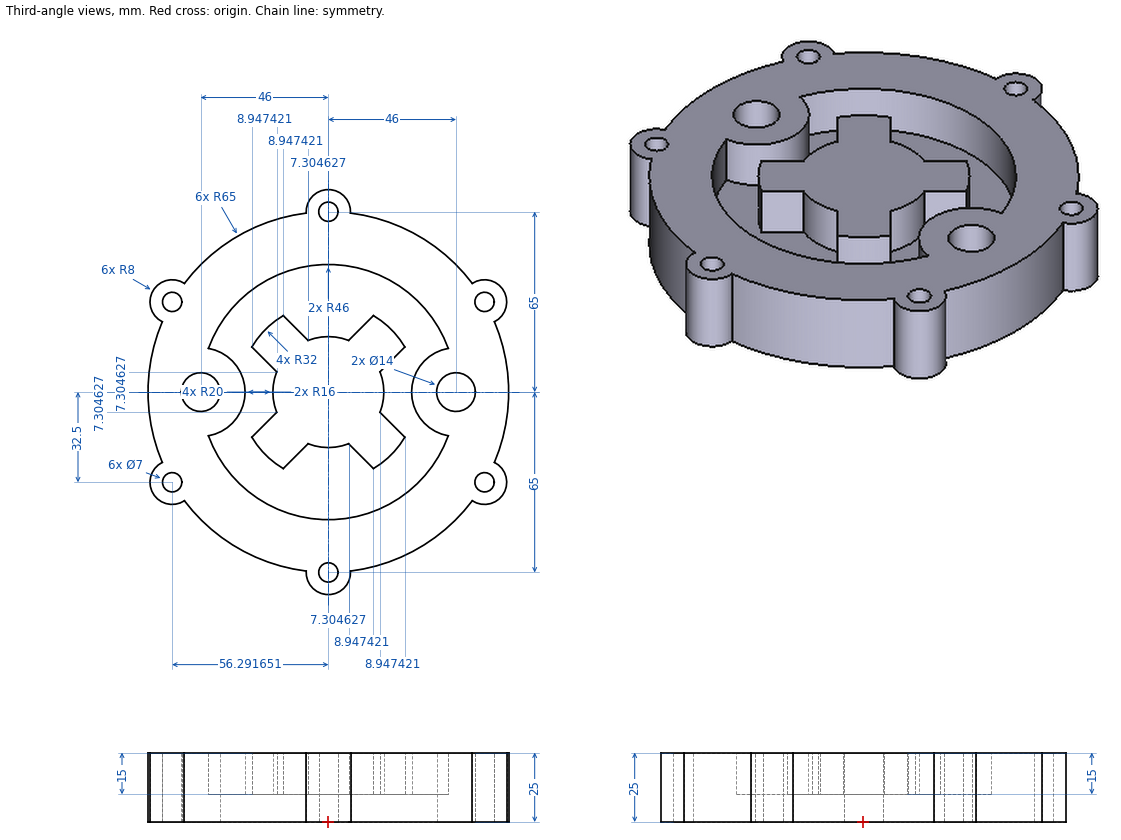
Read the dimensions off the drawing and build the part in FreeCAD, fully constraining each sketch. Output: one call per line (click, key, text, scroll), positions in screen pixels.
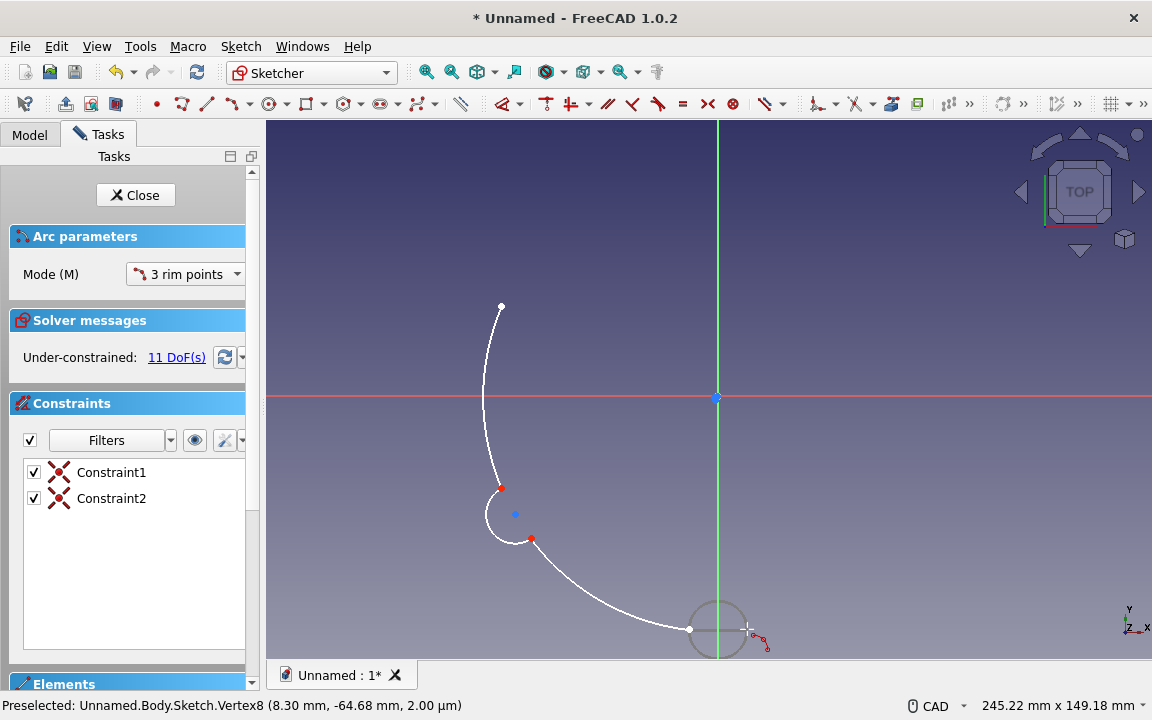
scroll(483, 376, down, 2)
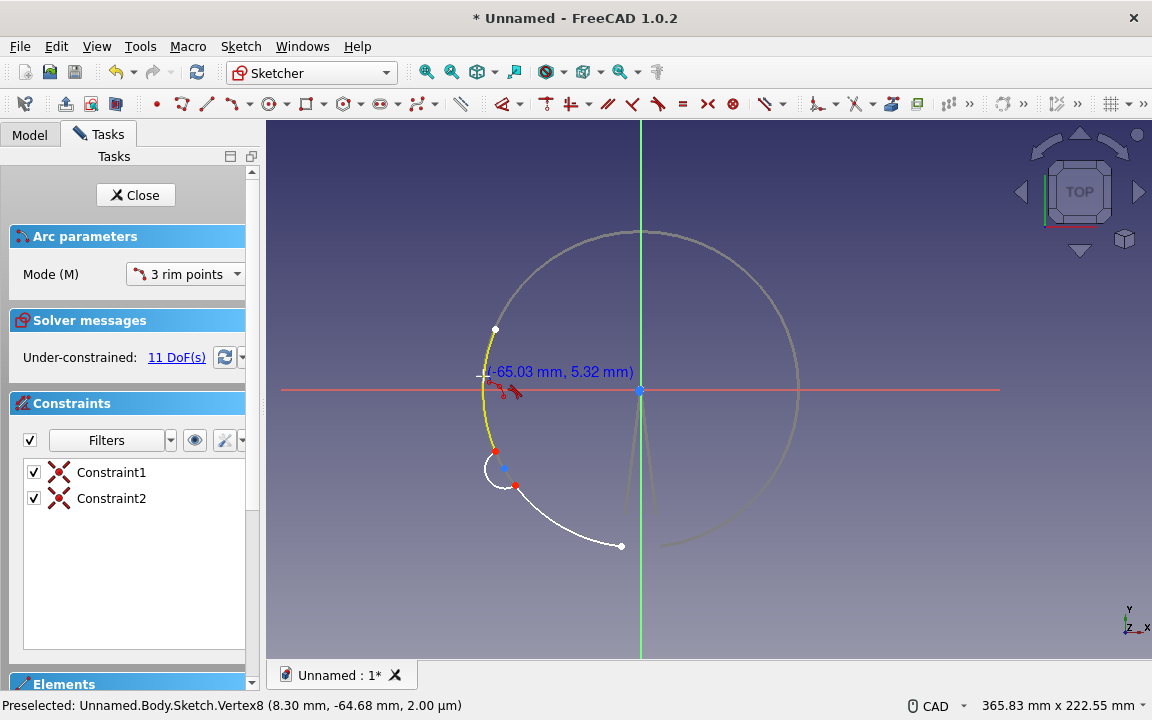
scroll(629, 563, up, 2)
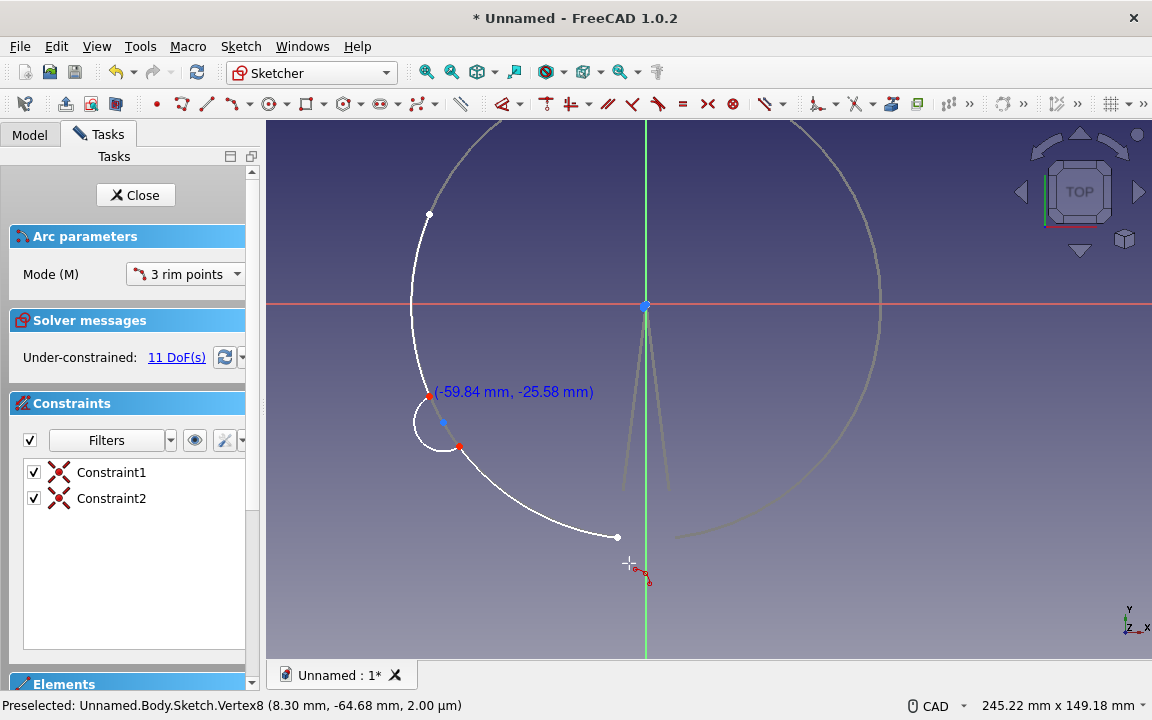
click(629, 562)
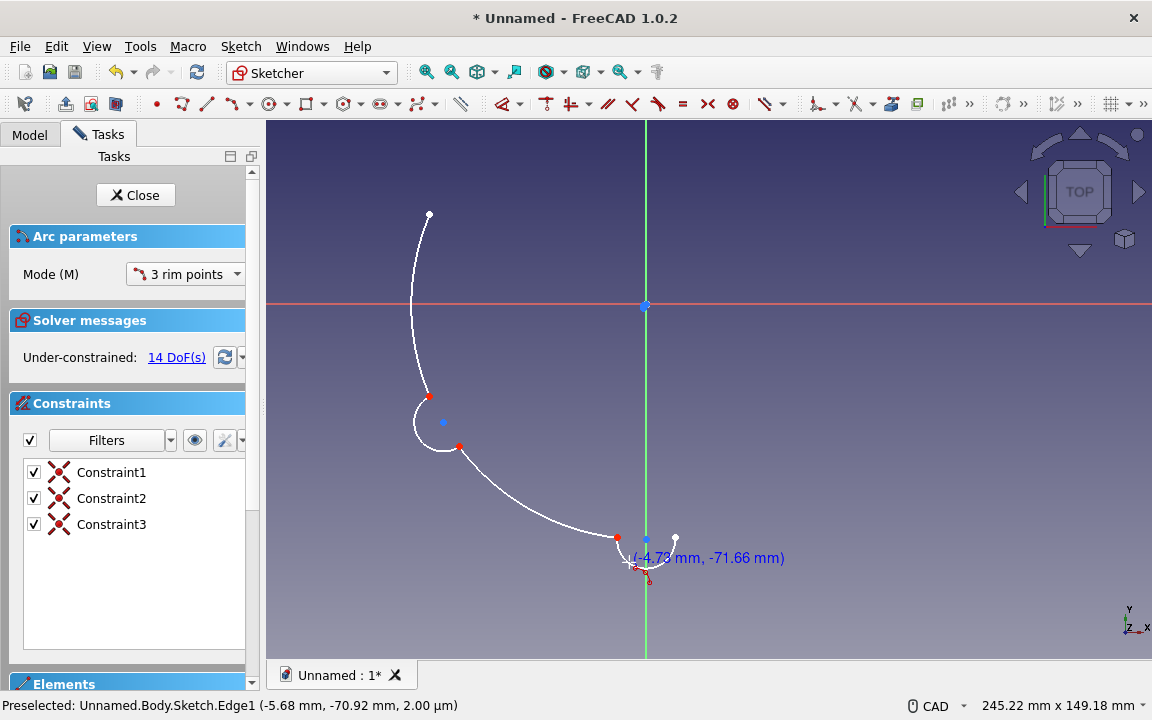
click(675, 538)
click(833, 446)
click(764, 507)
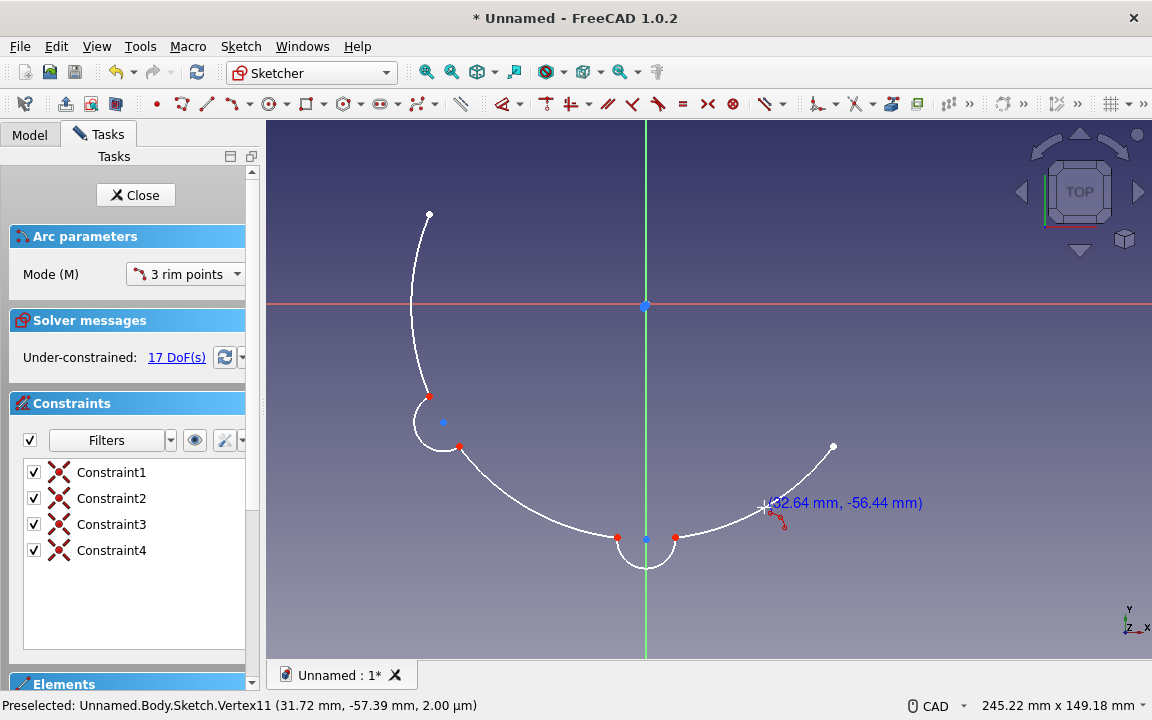
click(833, 447)
click(862, 396)
click(874, 436)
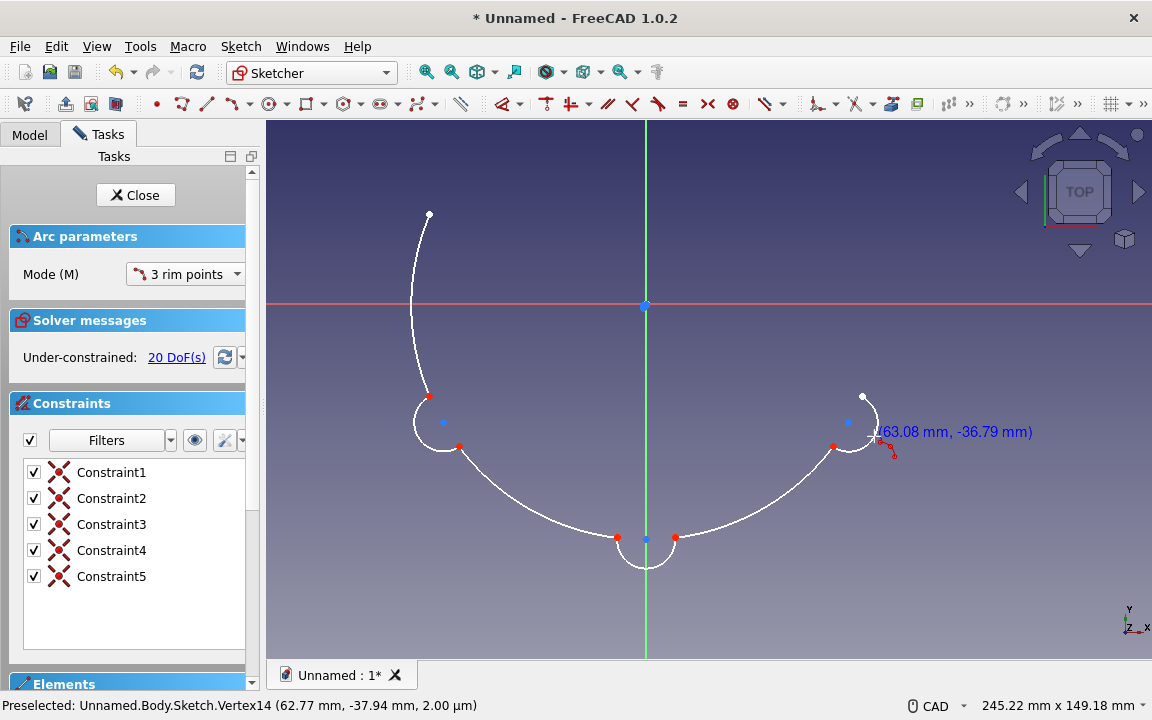
click(862, 397)
click(862, 213)
click(880, 323)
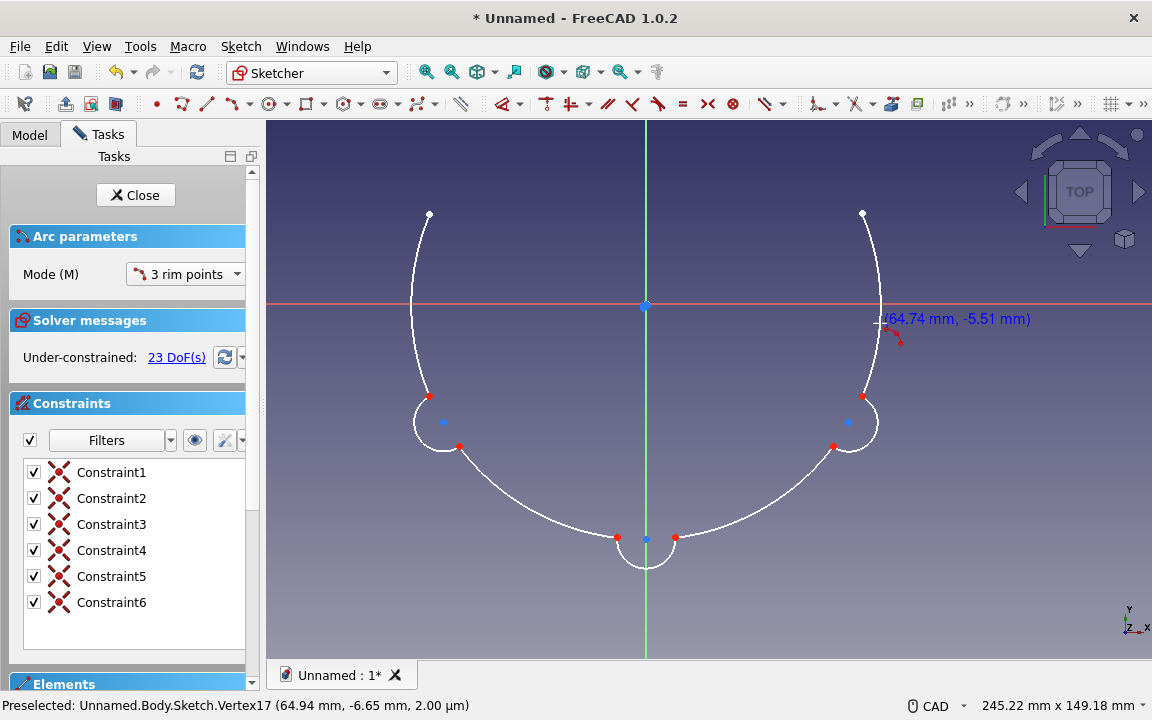
click(862, 214)
click(833, 163)
click(874, 172)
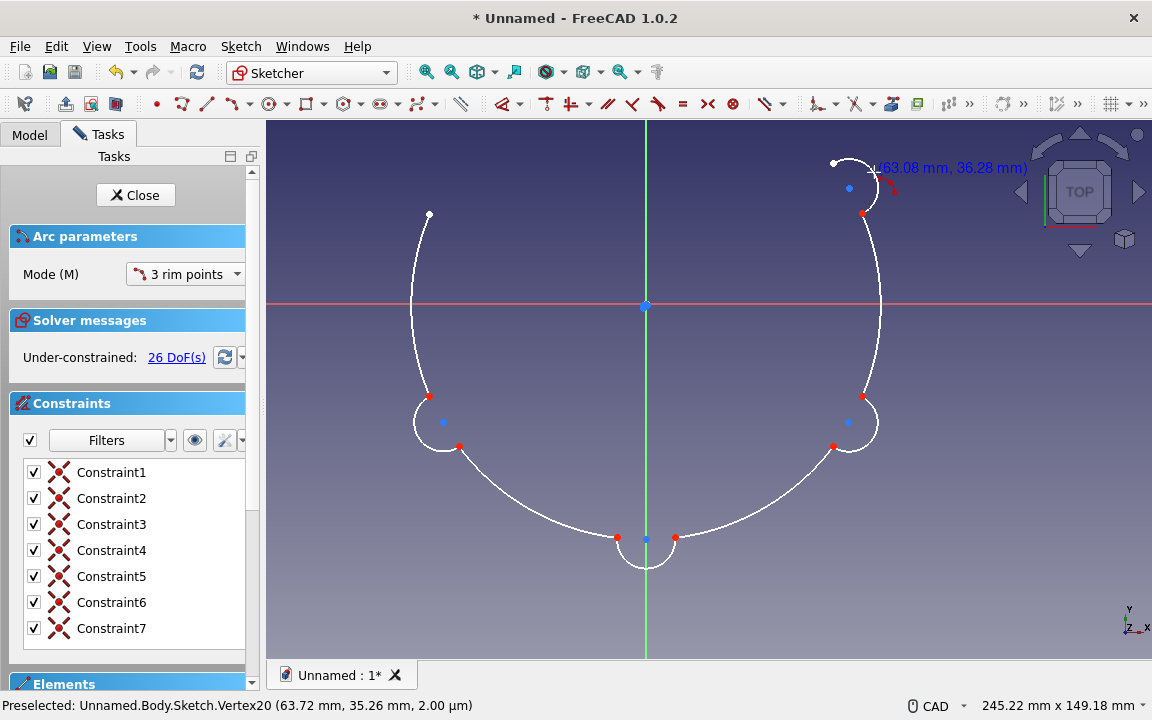
click(833, 164)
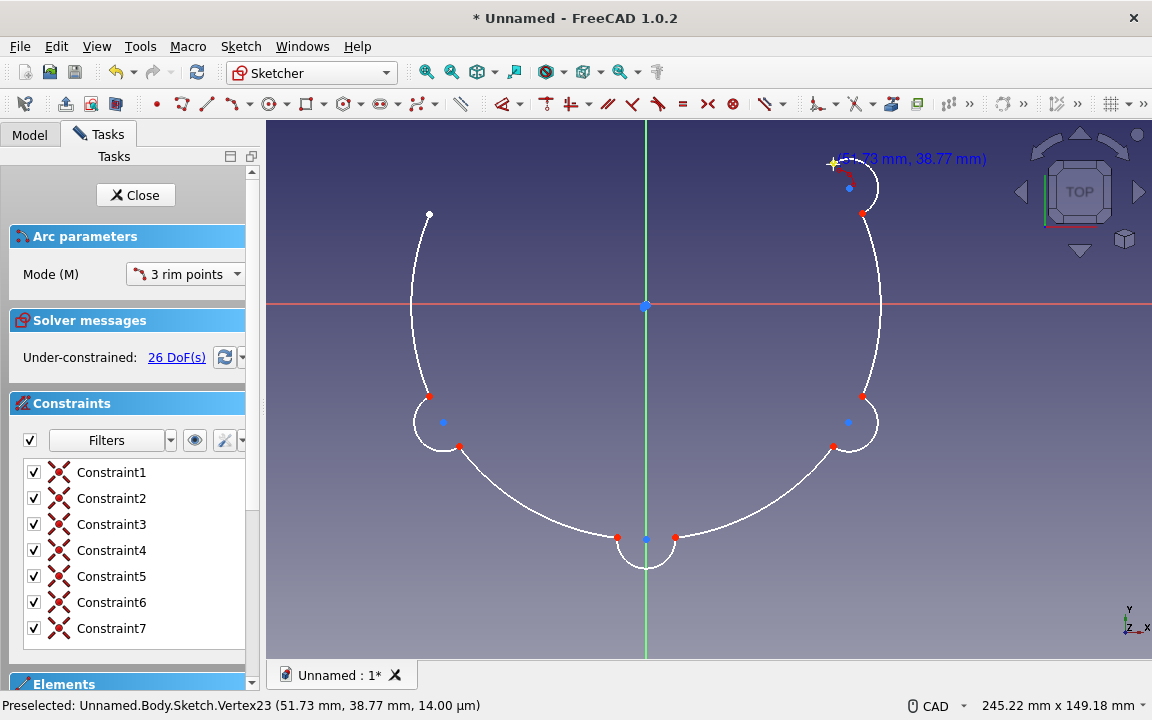
scroll(629, 563, down, 2)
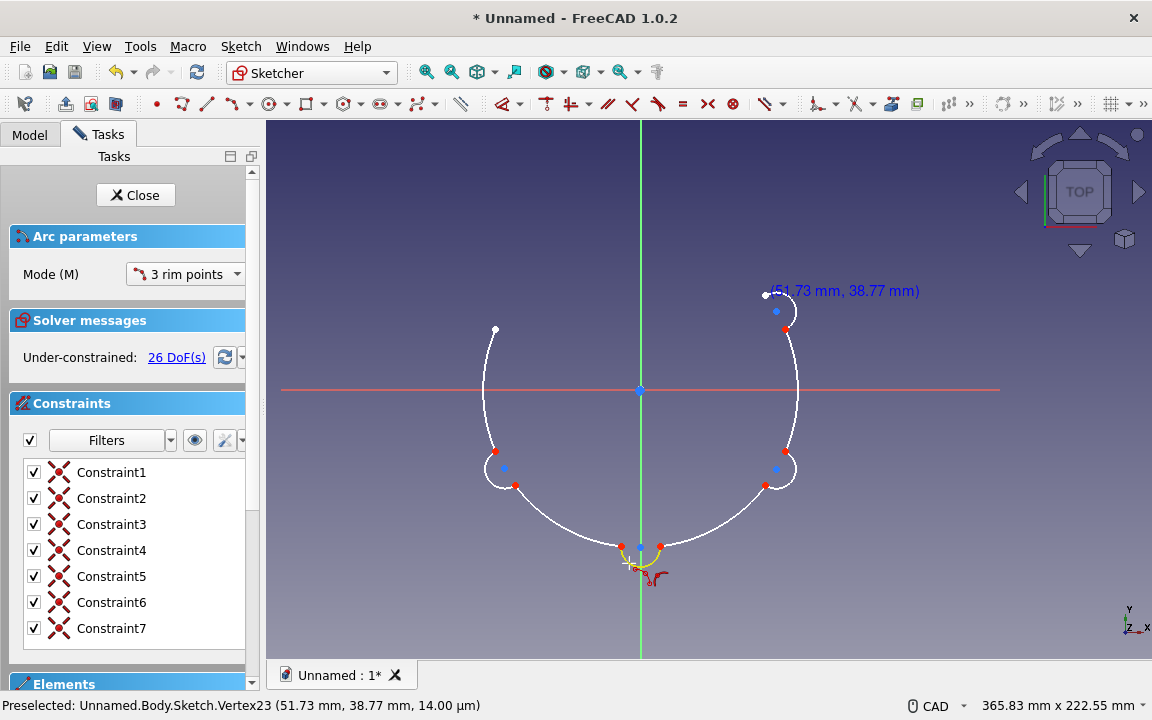
click(660, 233)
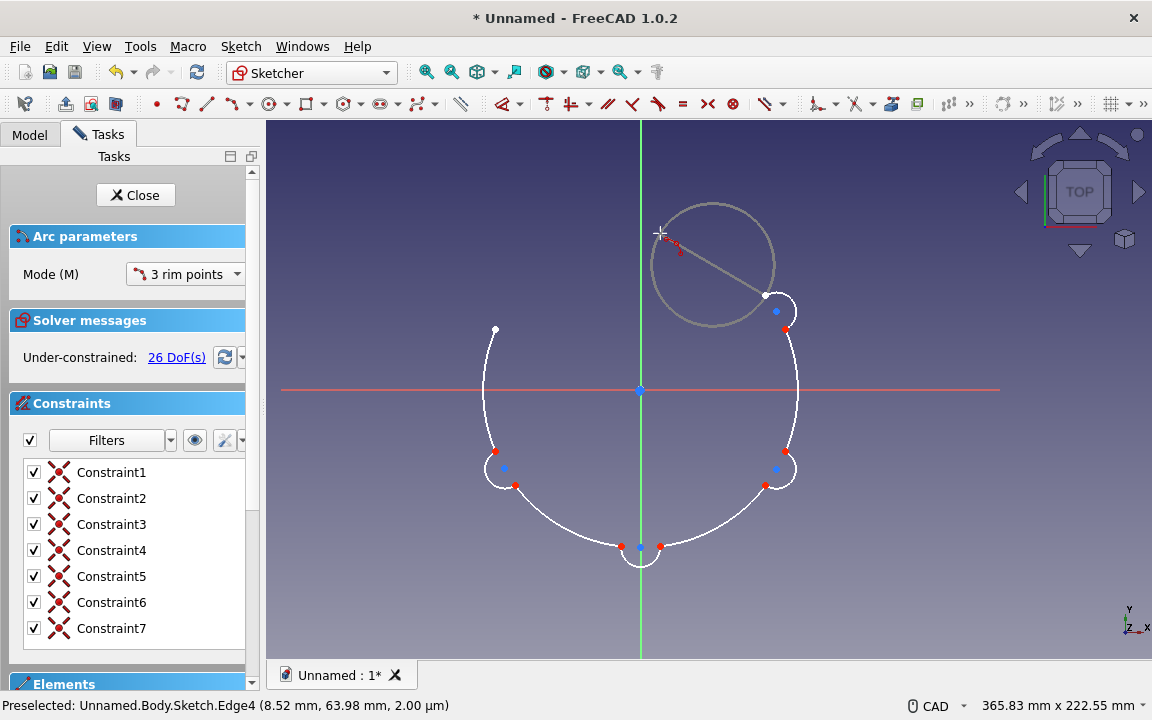
scroll(719, 253, up, 2)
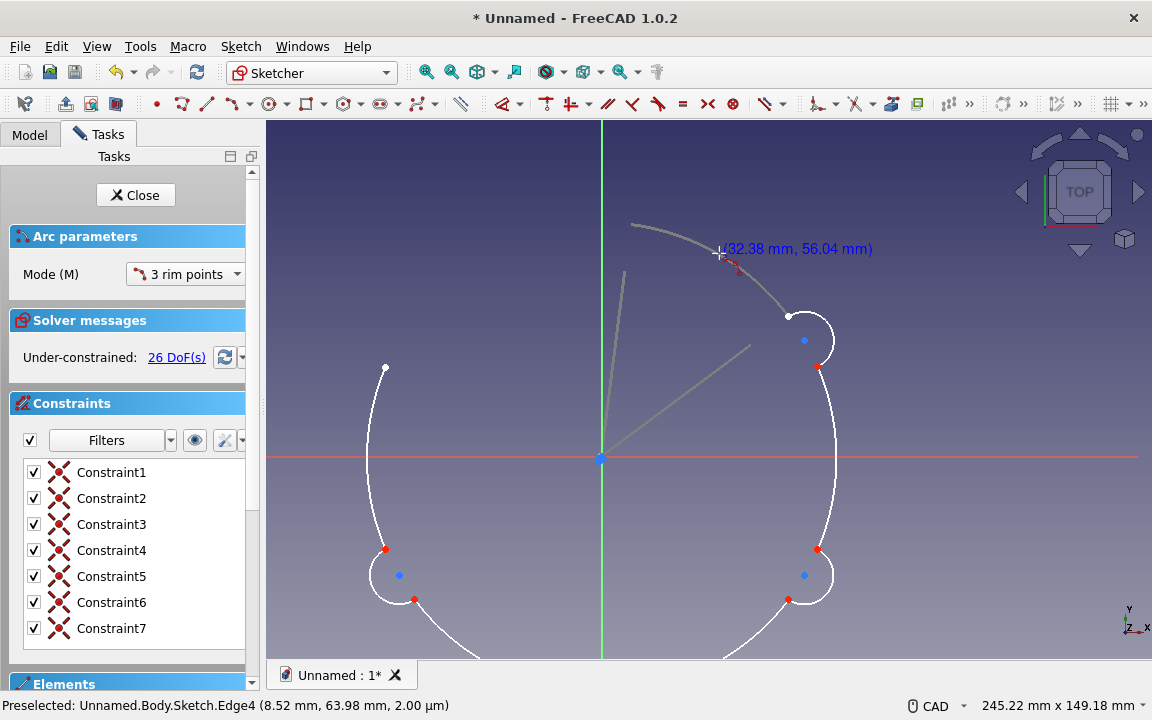
click(719, 253)